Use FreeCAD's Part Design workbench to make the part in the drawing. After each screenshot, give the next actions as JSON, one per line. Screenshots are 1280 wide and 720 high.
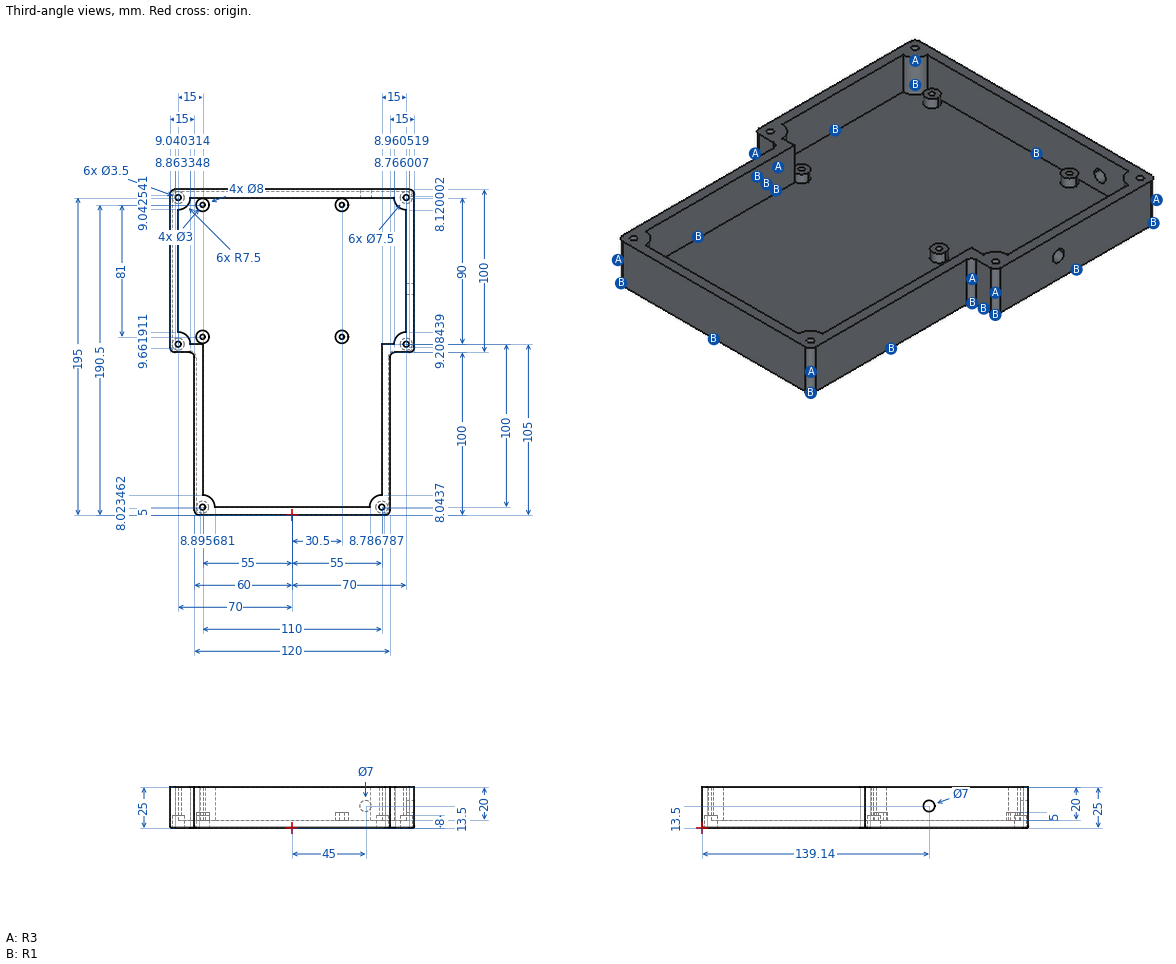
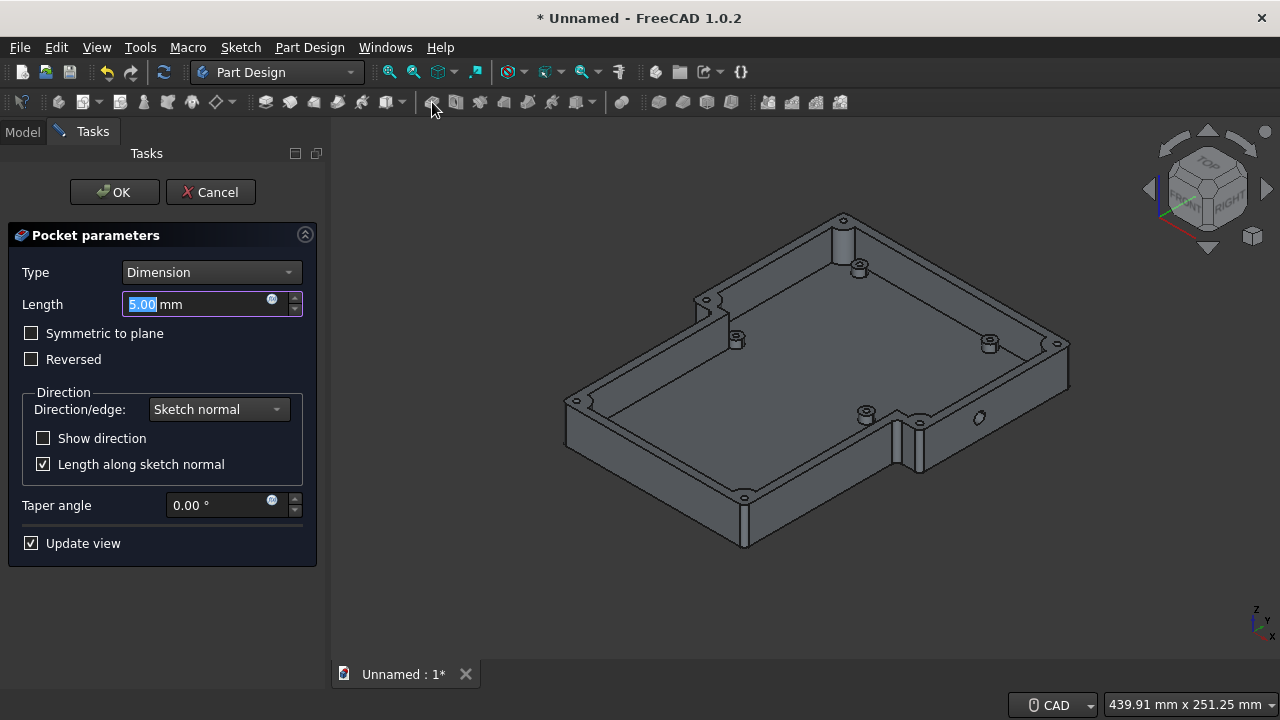
{"action": "left_click", "coordinate": [212, 272]}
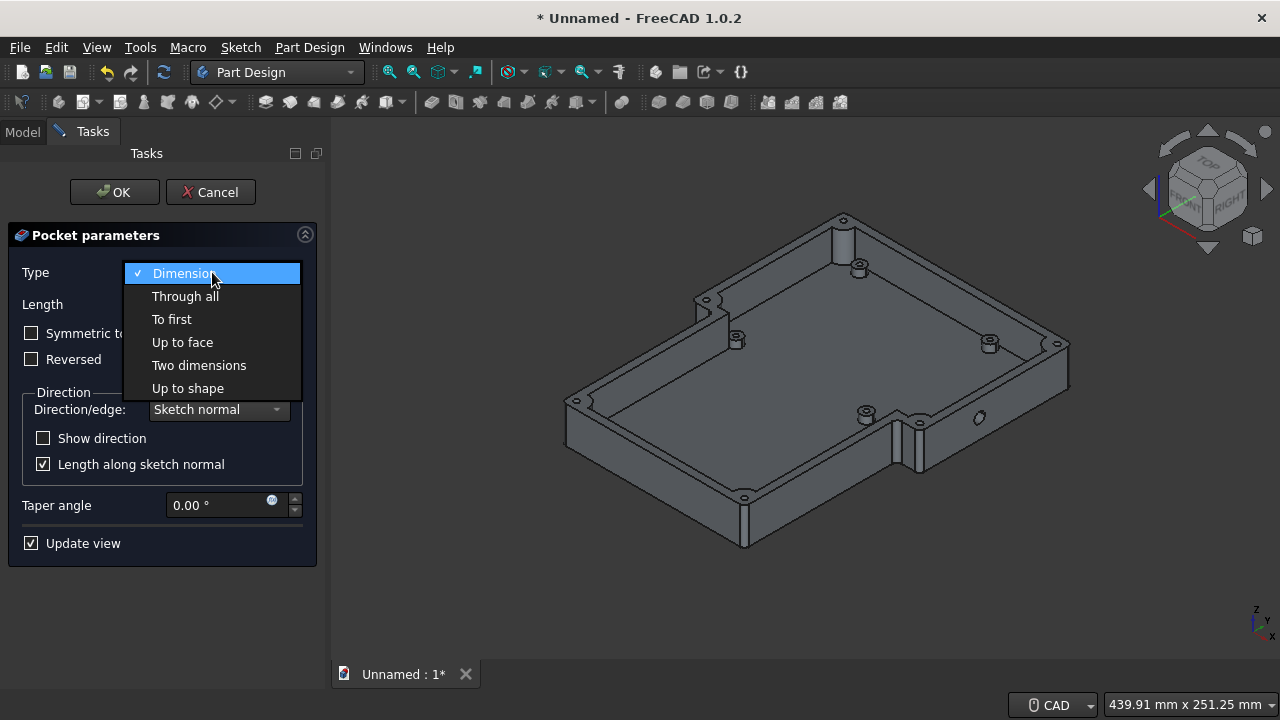
{"action": "left_click", "coordinate": [212, 320]}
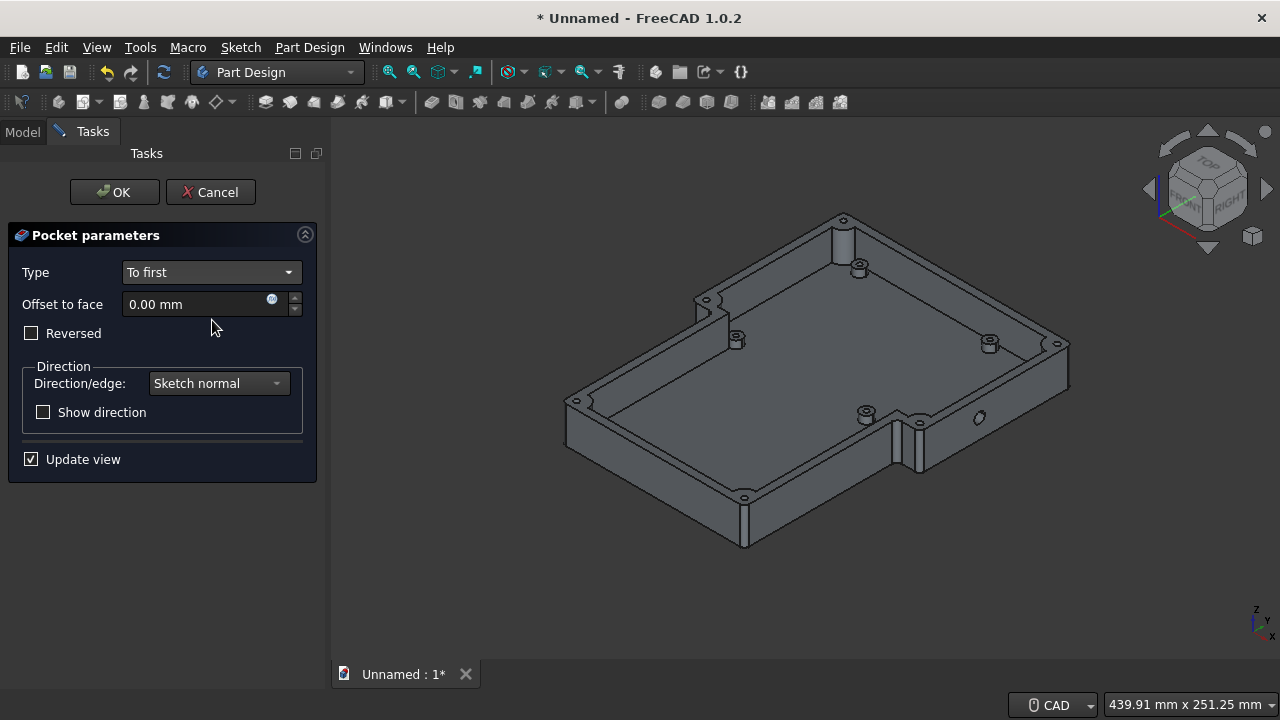
{"action": "left_click", "coordinate": [115, 192]}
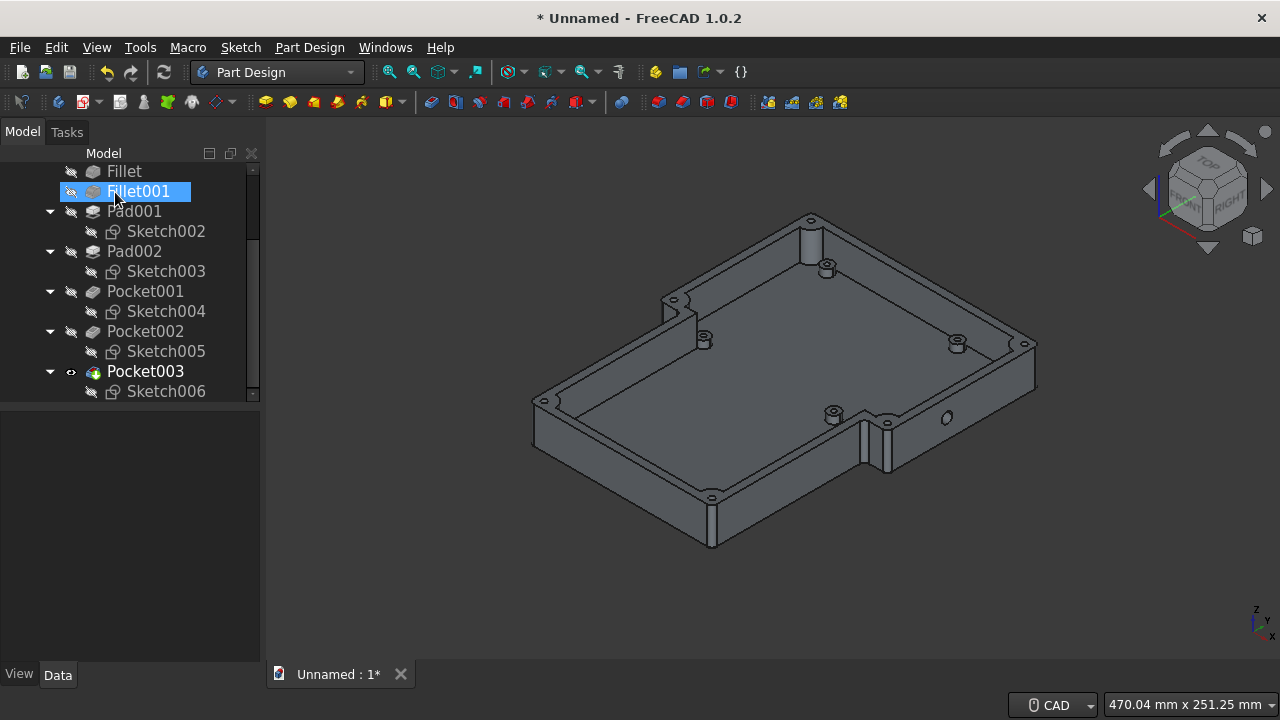
{"action": "key", "text": "4"}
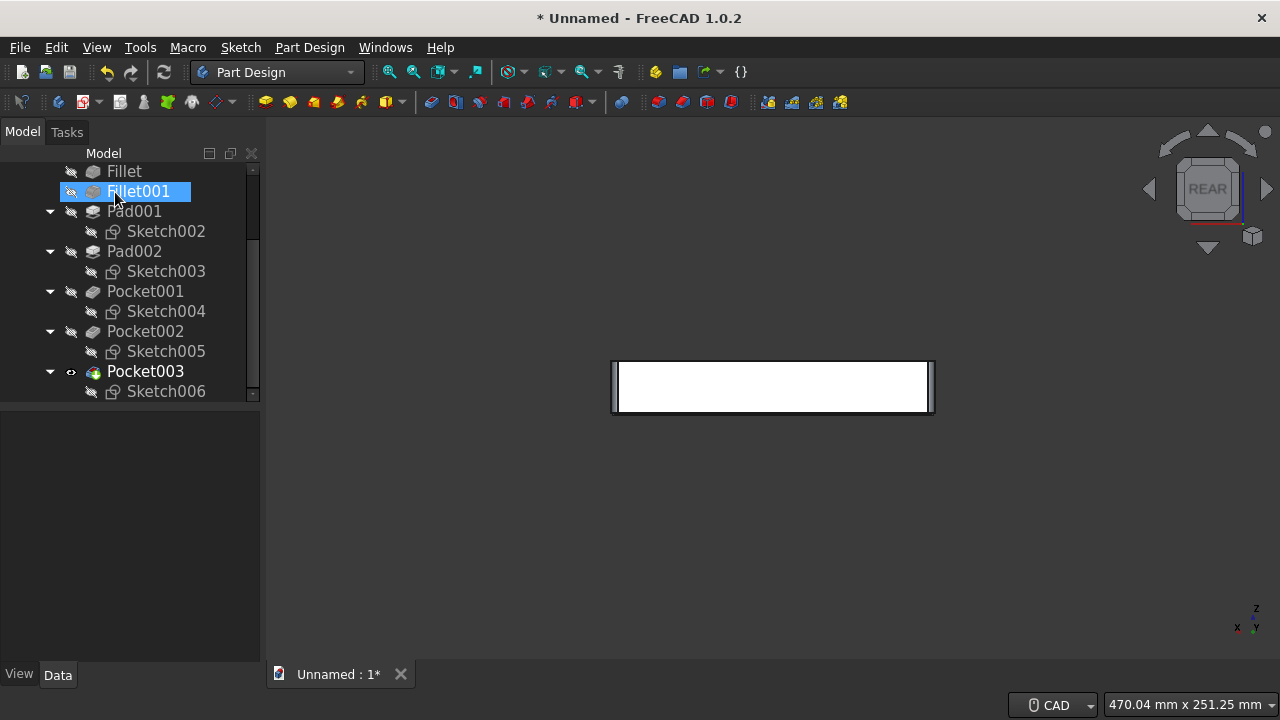
{"action": "key", "text": "v f"}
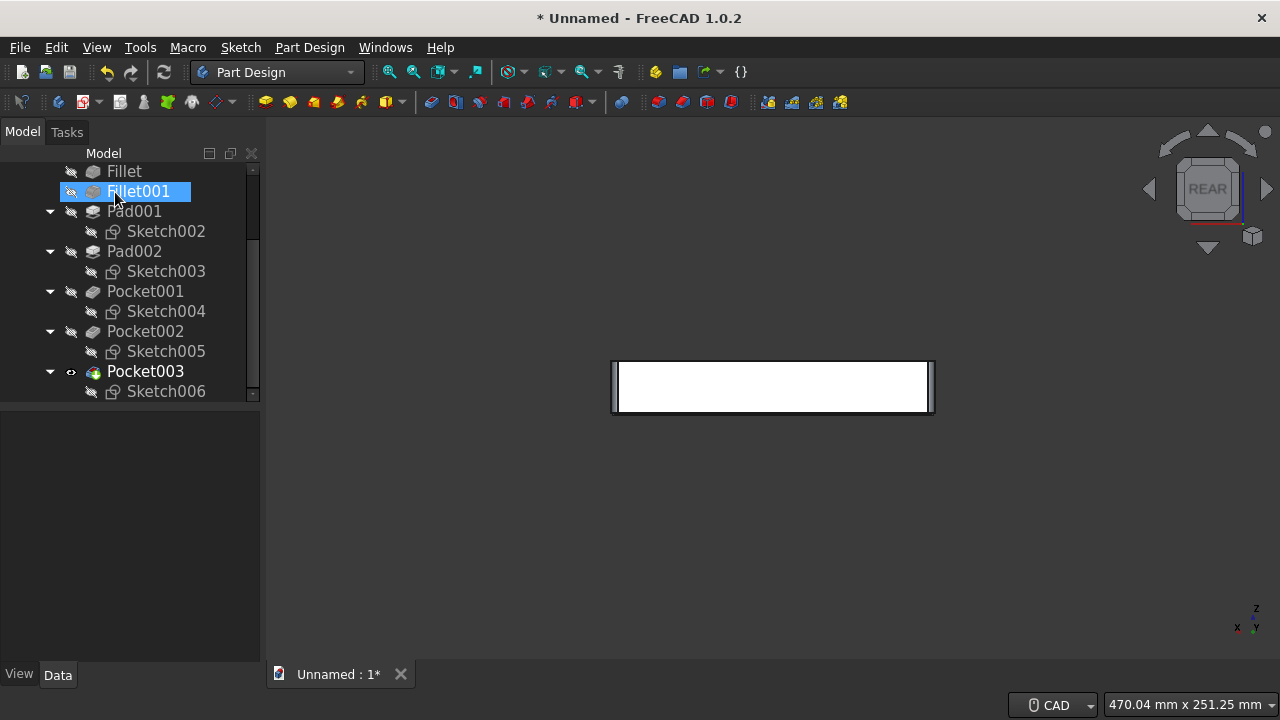
{"action": "left_click", "coordinate": [684, 386]}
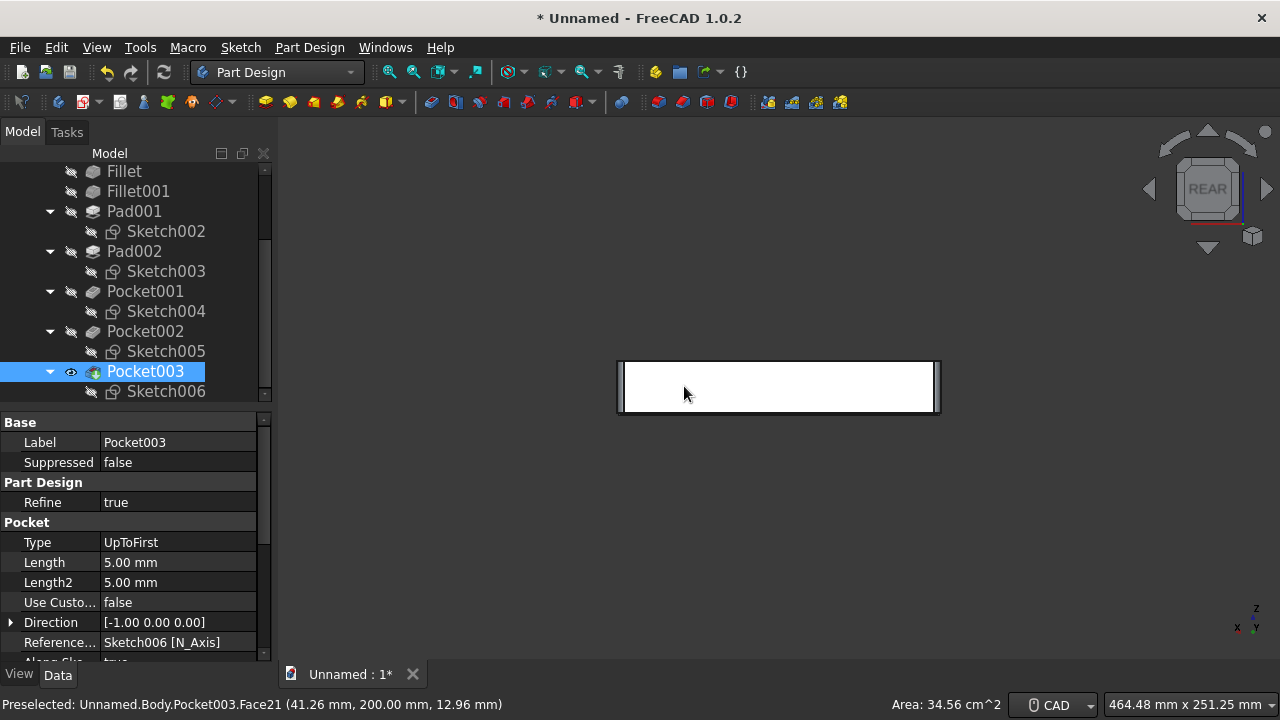
{"action": "left_click", "coordinate": [84, 102]}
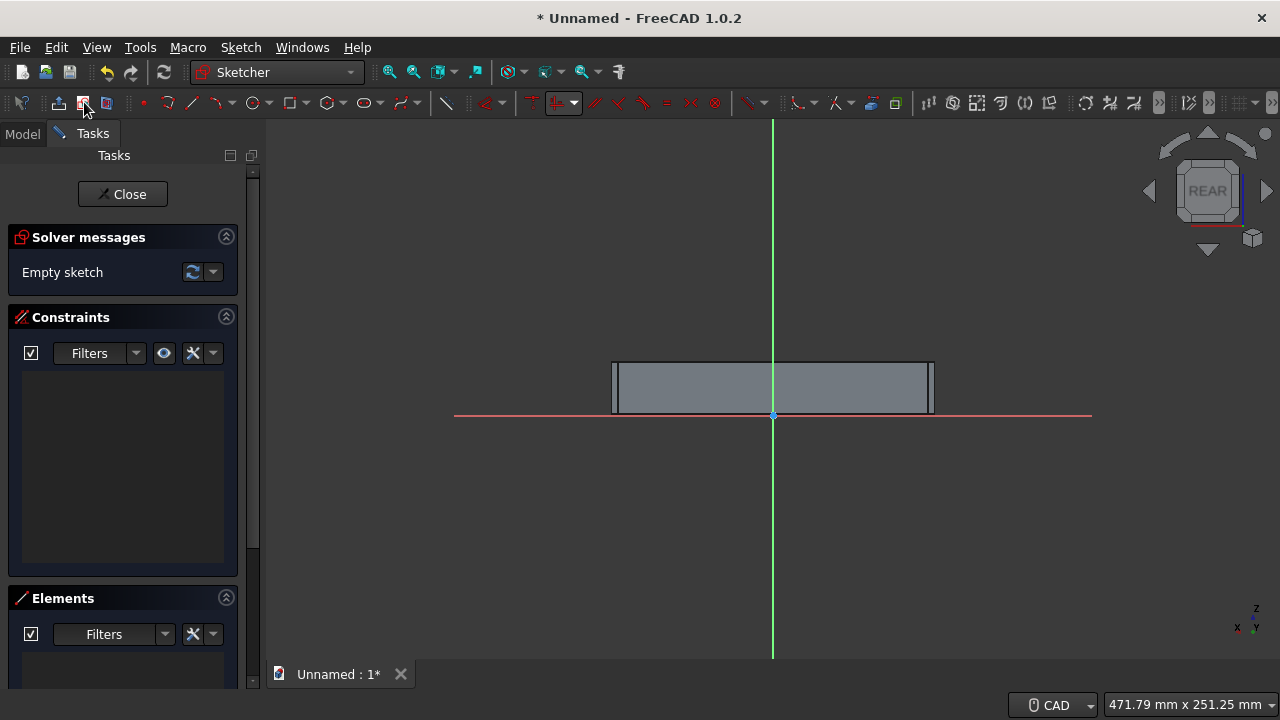
{"action": "scroll", "coordinate": [675, 387], "scroll_direction": "up", "scroll_amount": 15}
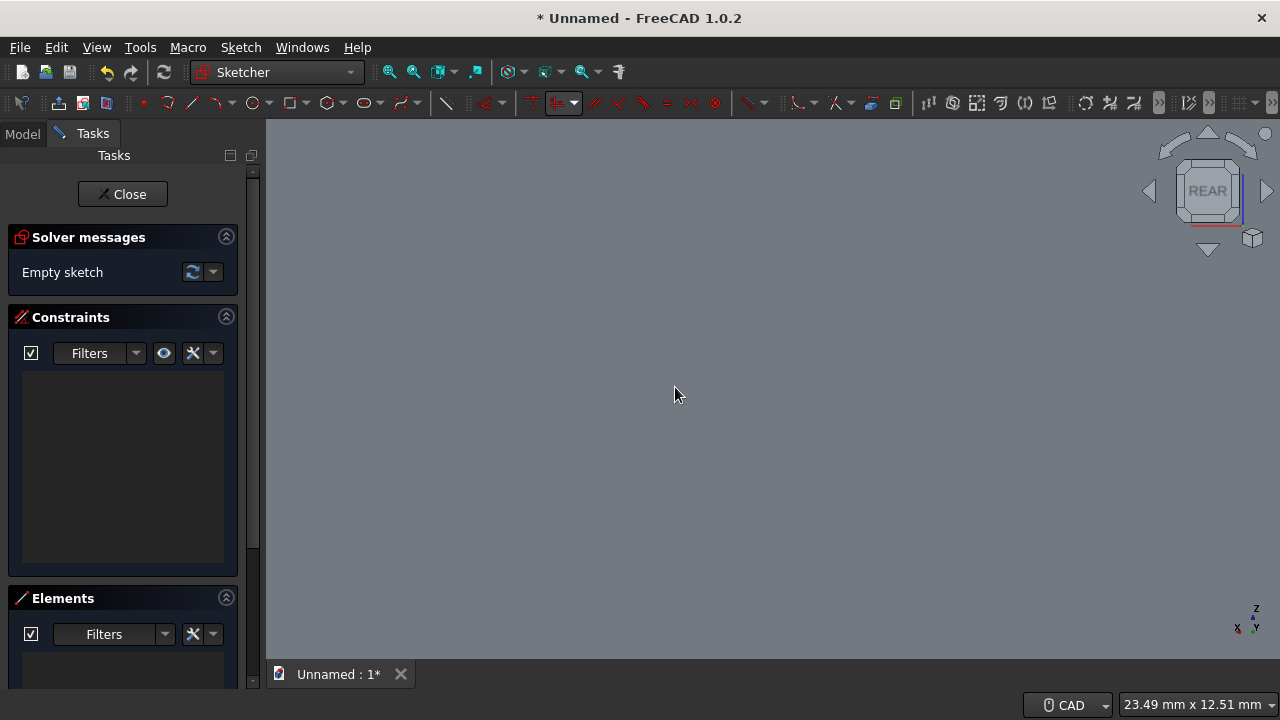
{"action": "key", "text": "g c"}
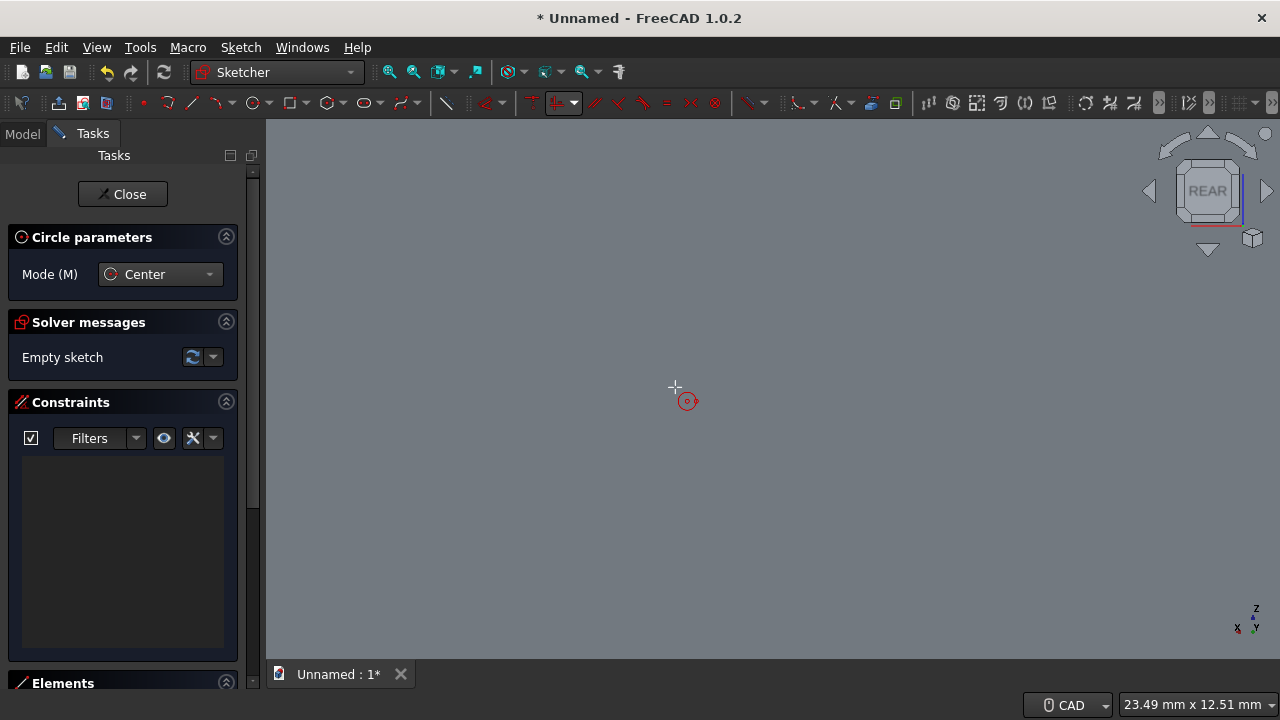
{"action": "left_click", "coordinate": [693, 375]}
{"action": "mouse_move", "coordinate": [800, 268]}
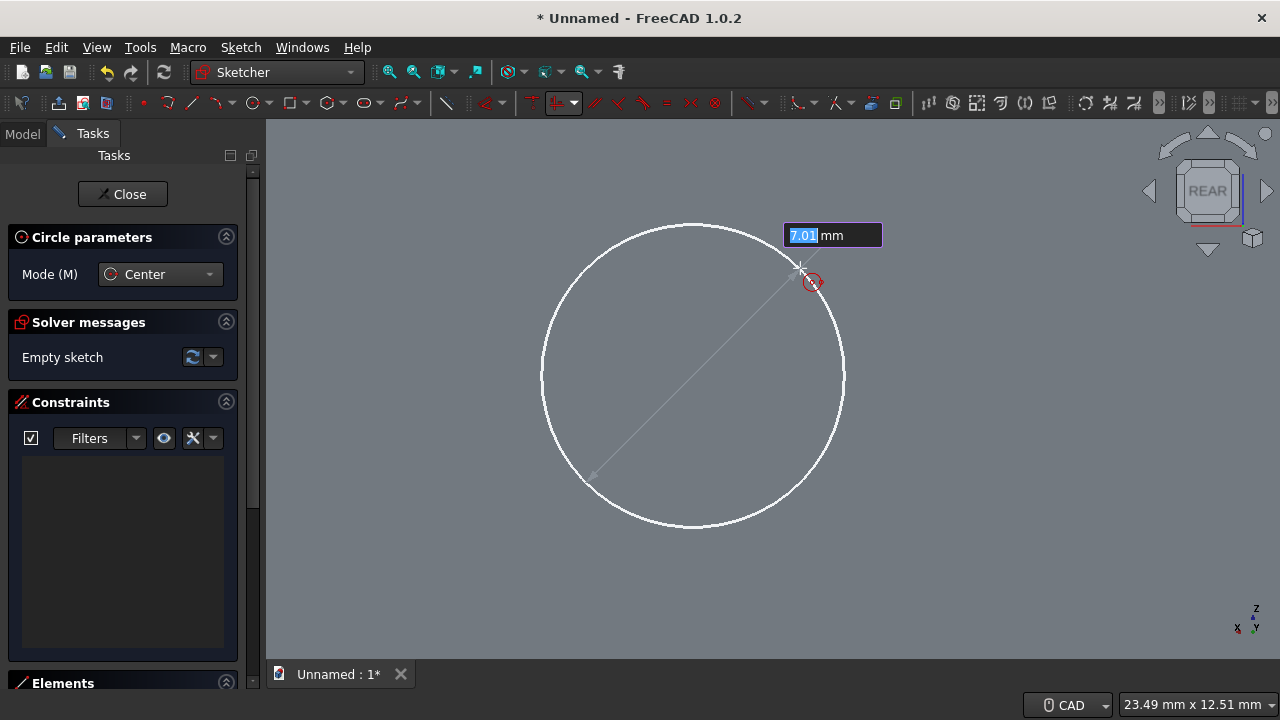
{"action": "type", "text": "7"}
{"action": "key", "text": "Return"}
{"action": "key", "text": "Escape"}